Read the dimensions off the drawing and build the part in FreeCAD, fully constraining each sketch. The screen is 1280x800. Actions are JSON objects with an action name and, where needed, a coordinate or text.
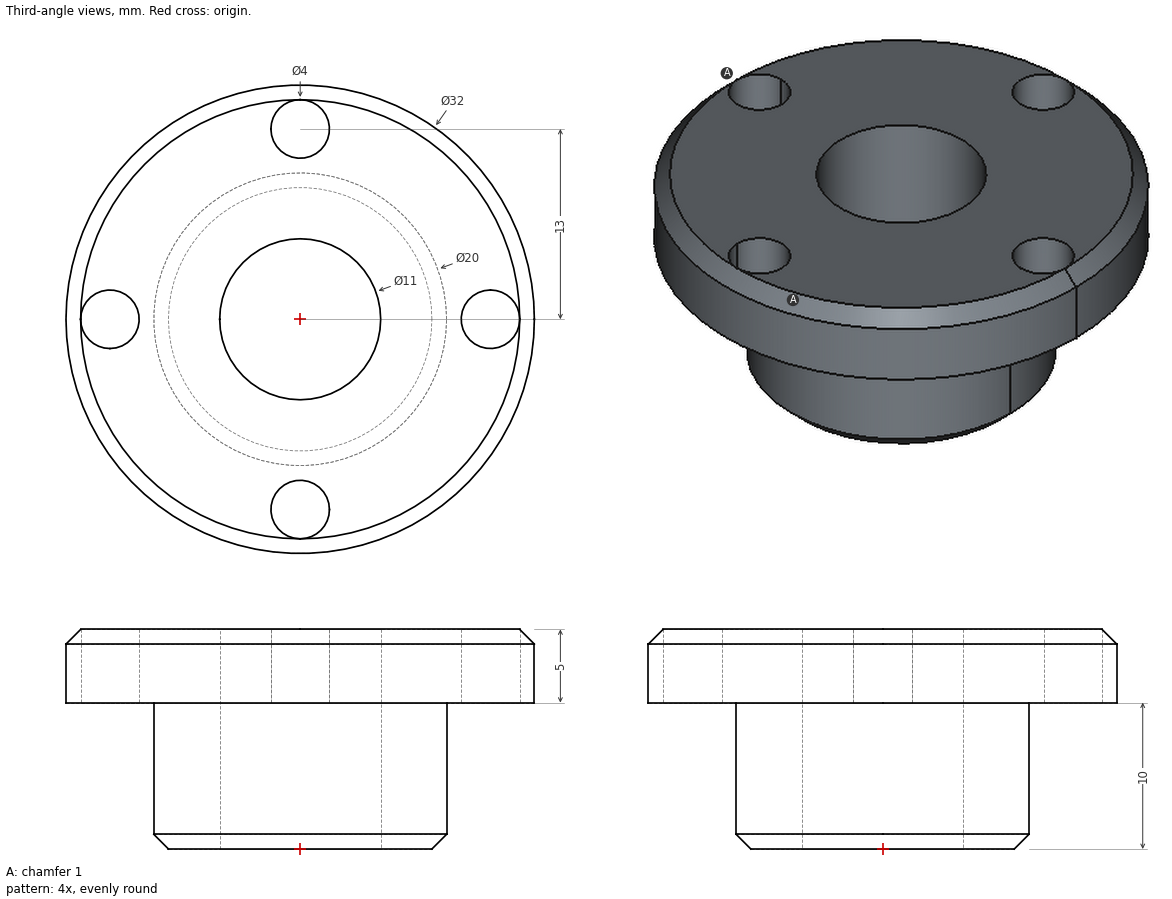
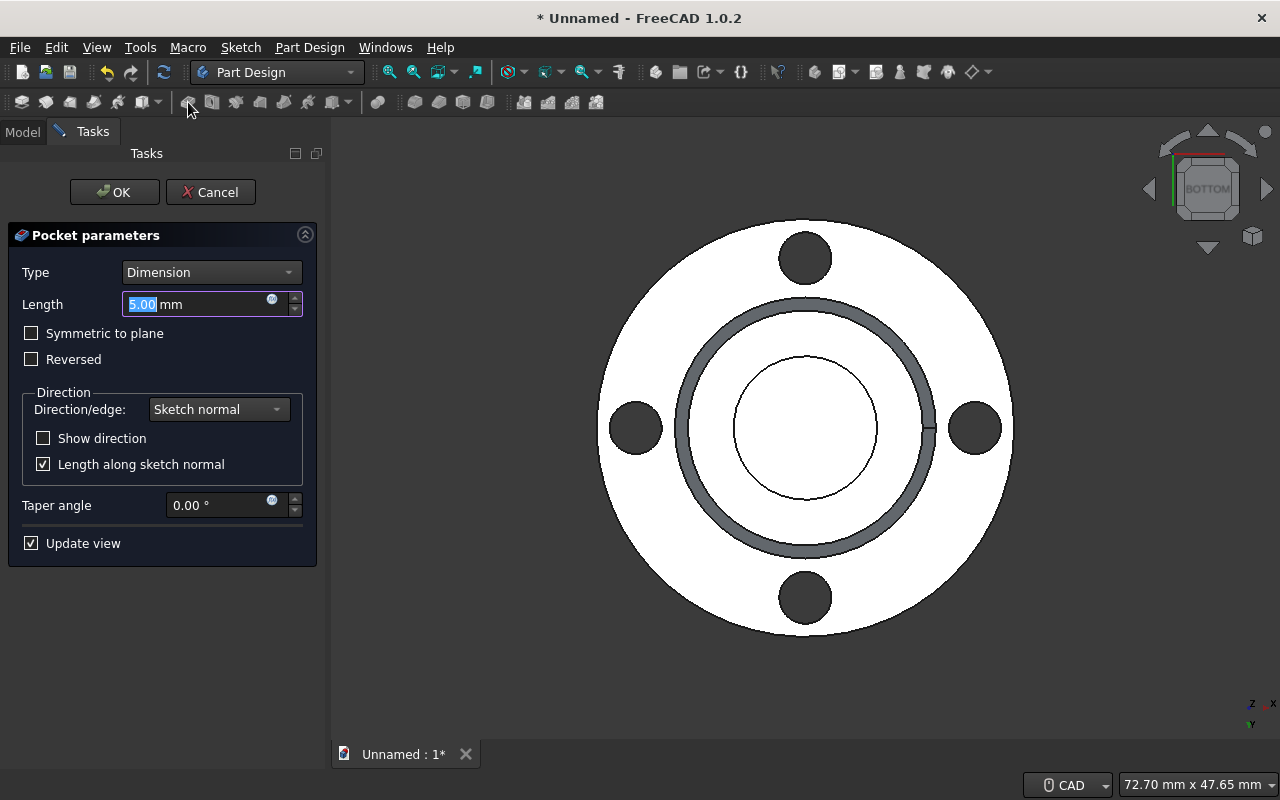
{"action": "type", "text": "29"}
{"action": "key", "text": "Tab"}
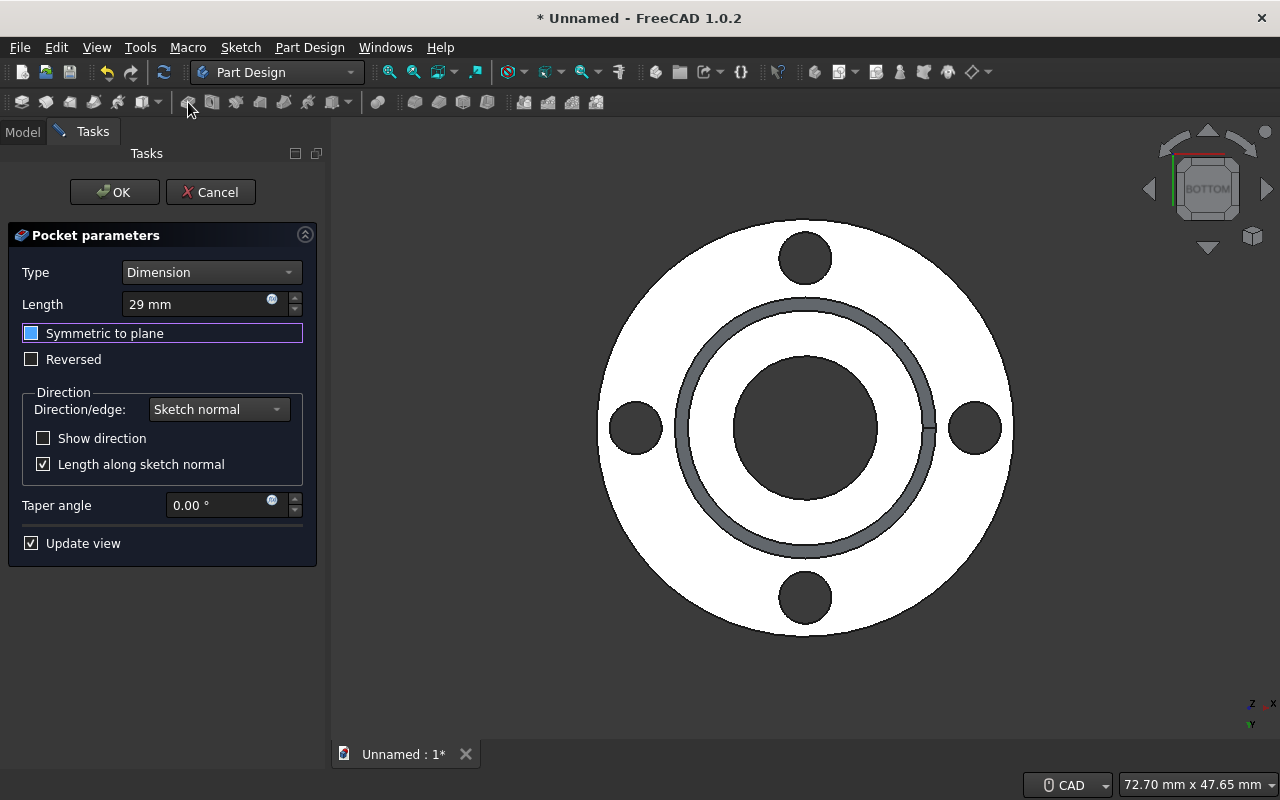
{"action": "left_click", "coordinate": [115, 192]}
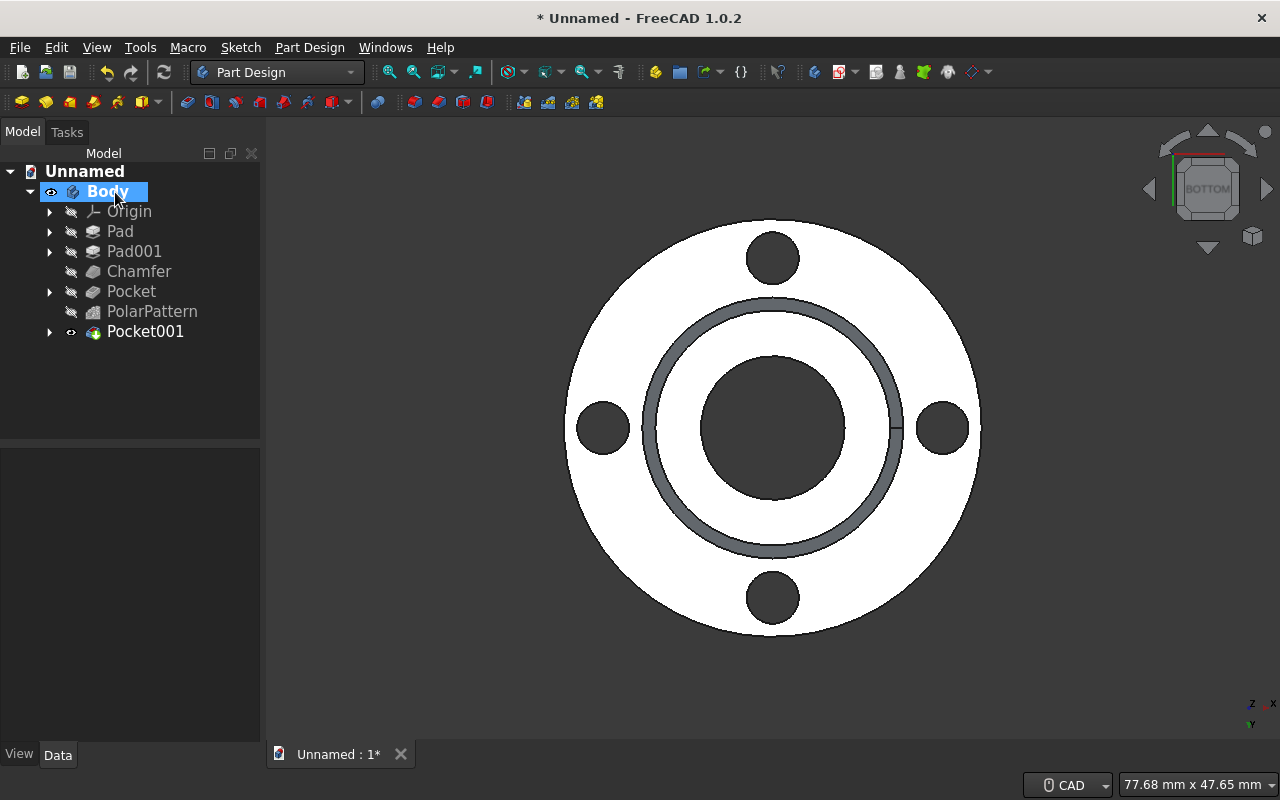
{"action": "key", "text": "0"}